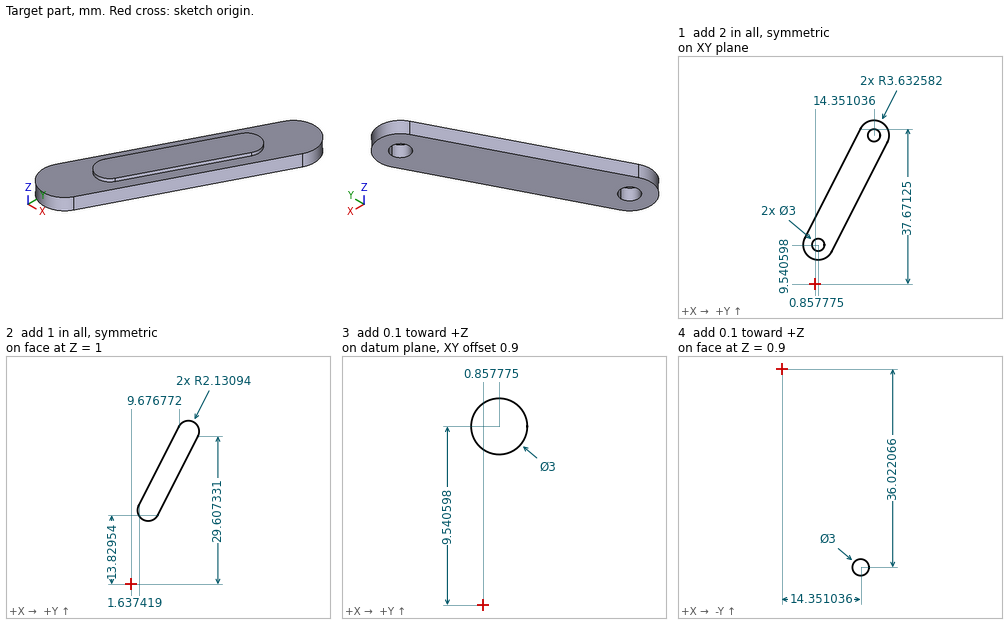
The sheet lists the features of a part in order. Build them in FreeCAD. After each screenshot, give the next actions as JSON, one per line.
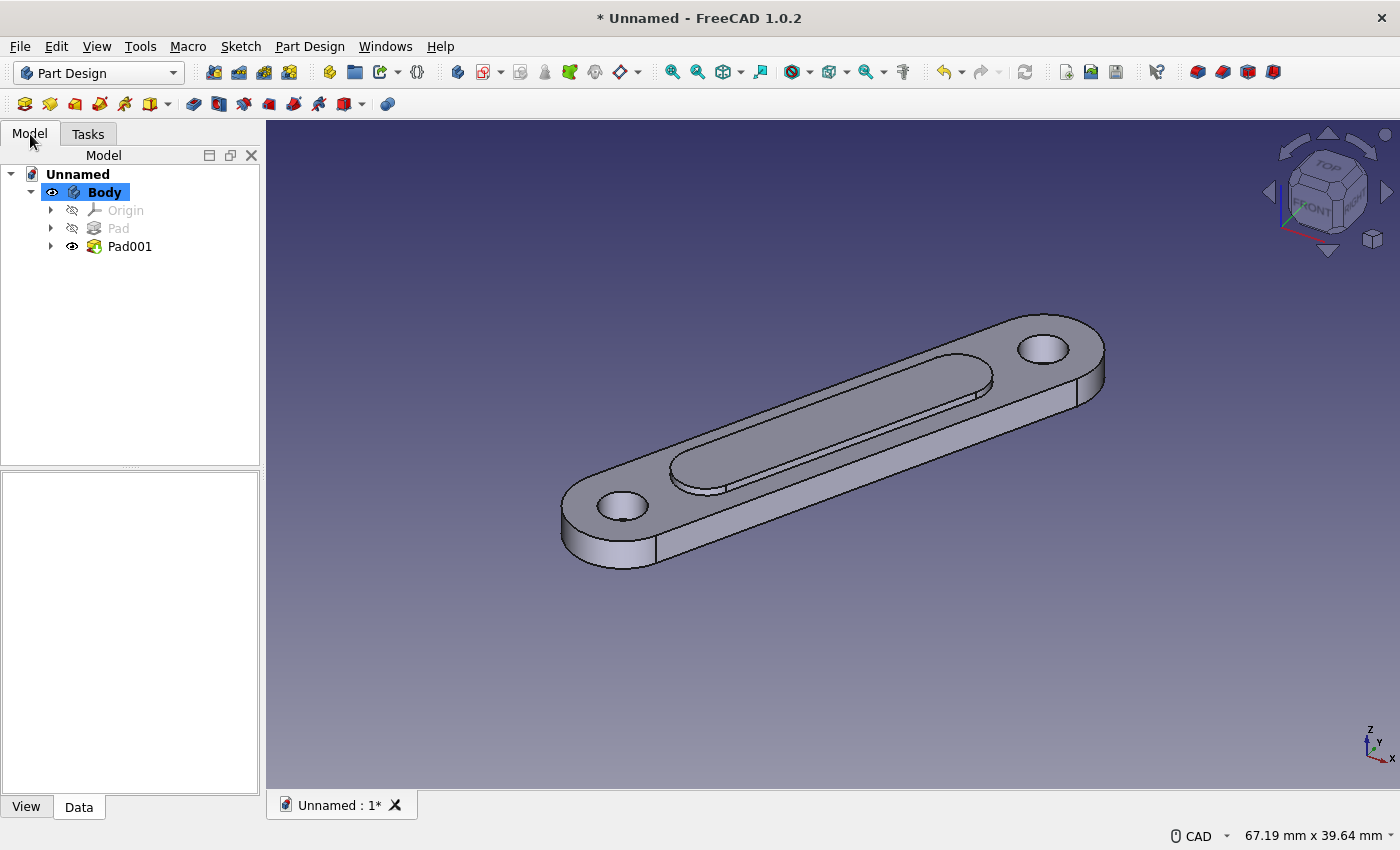
{"action": "left_click", "coordinate": [51, 210]}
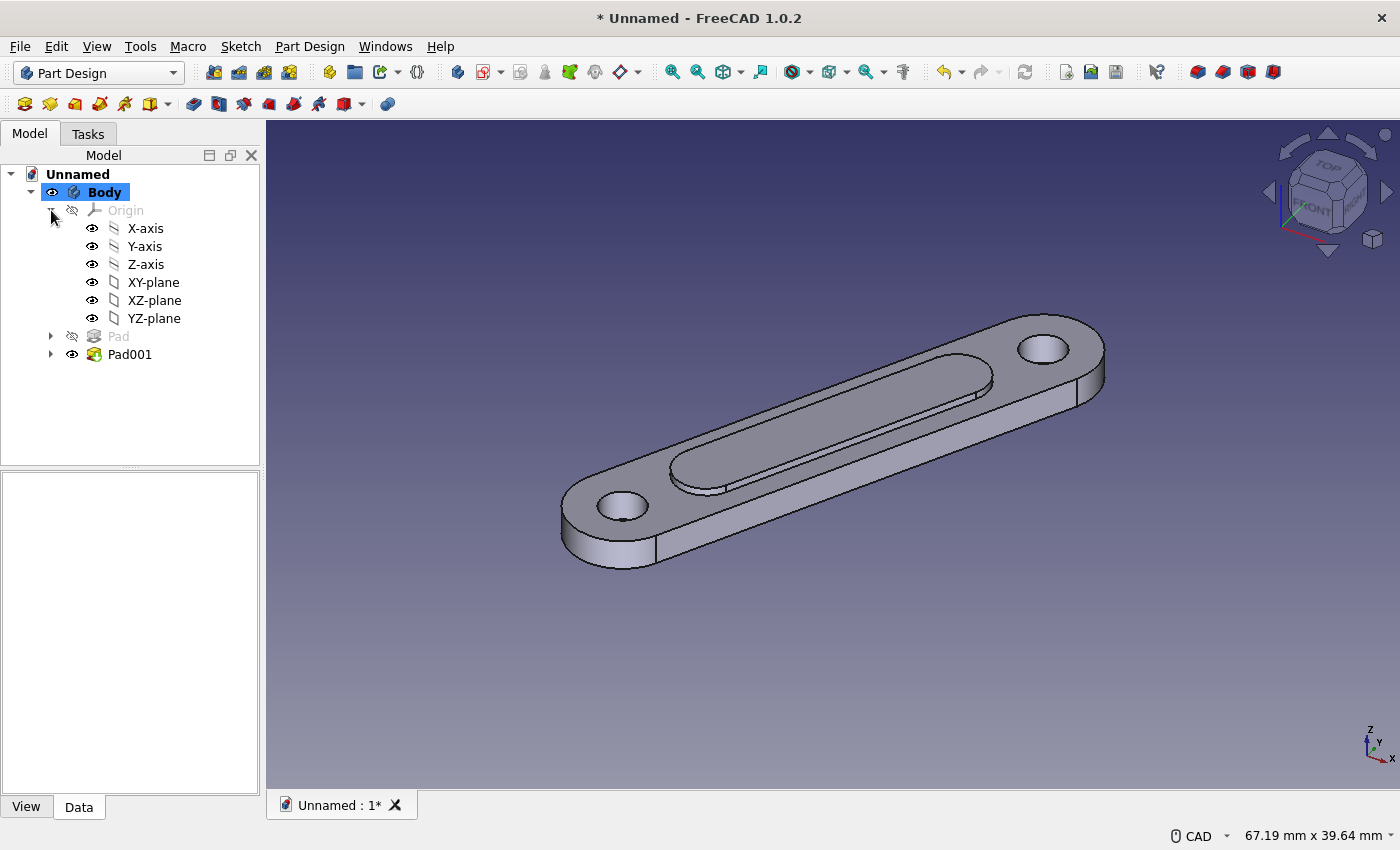
{"action": "left_click", "coordinate": [137, 282]}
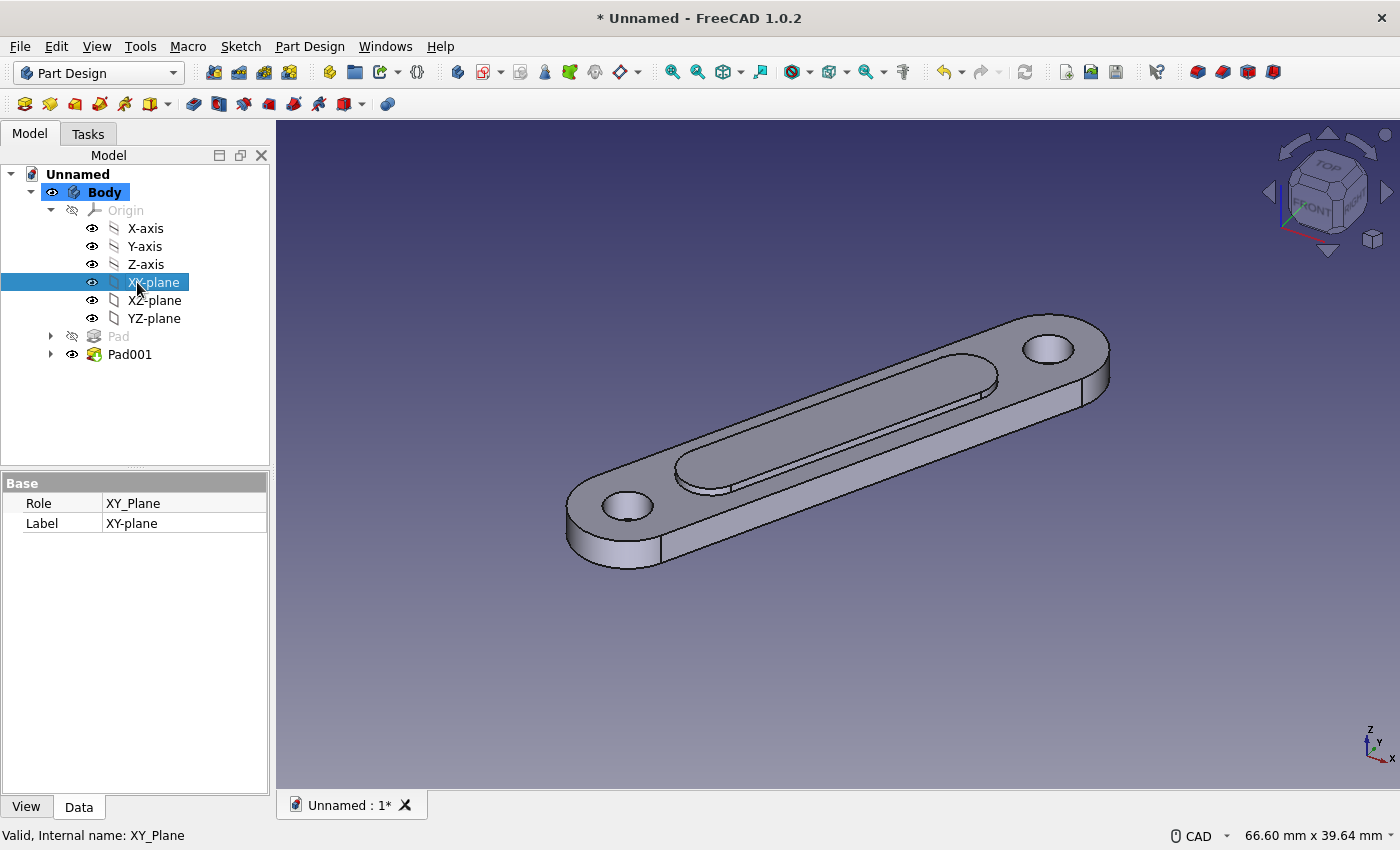
{"action": "left_click", "coordinate": [620, 72]}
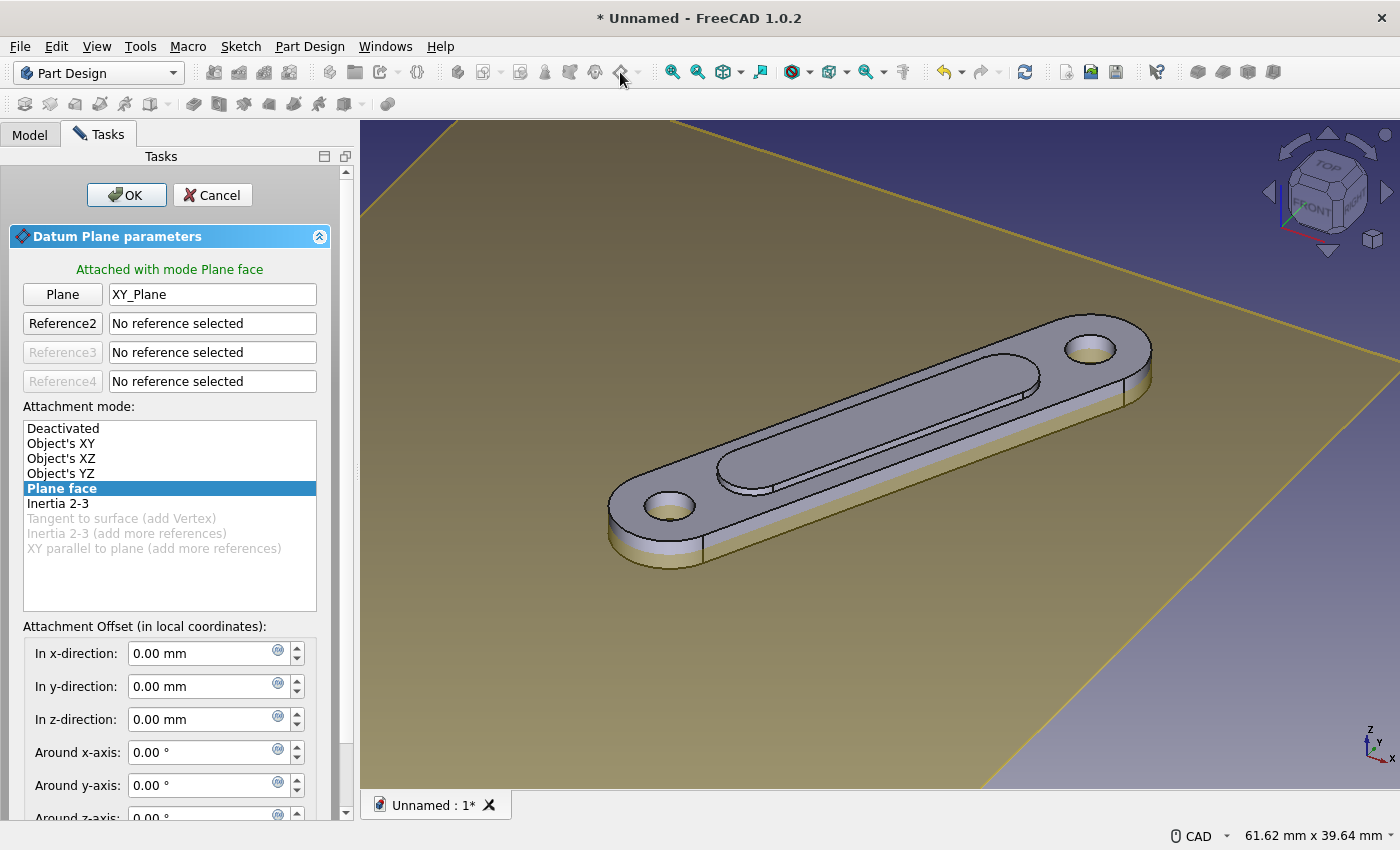
{"action": "triple_click", "coordinate": [210, 720]}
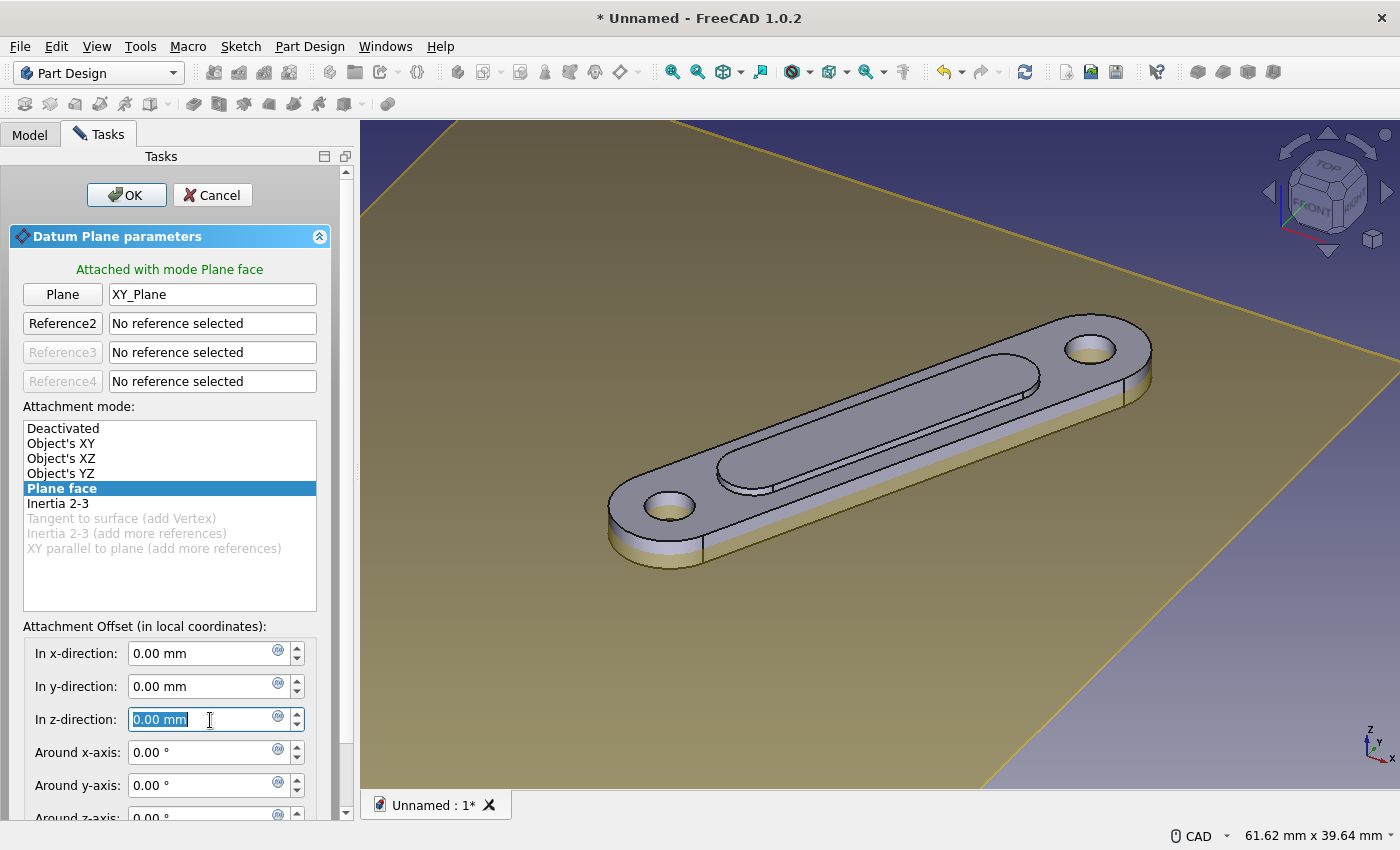
{"action": "type", "text": "0.9"}
{"action": "key", "text": "Tab"}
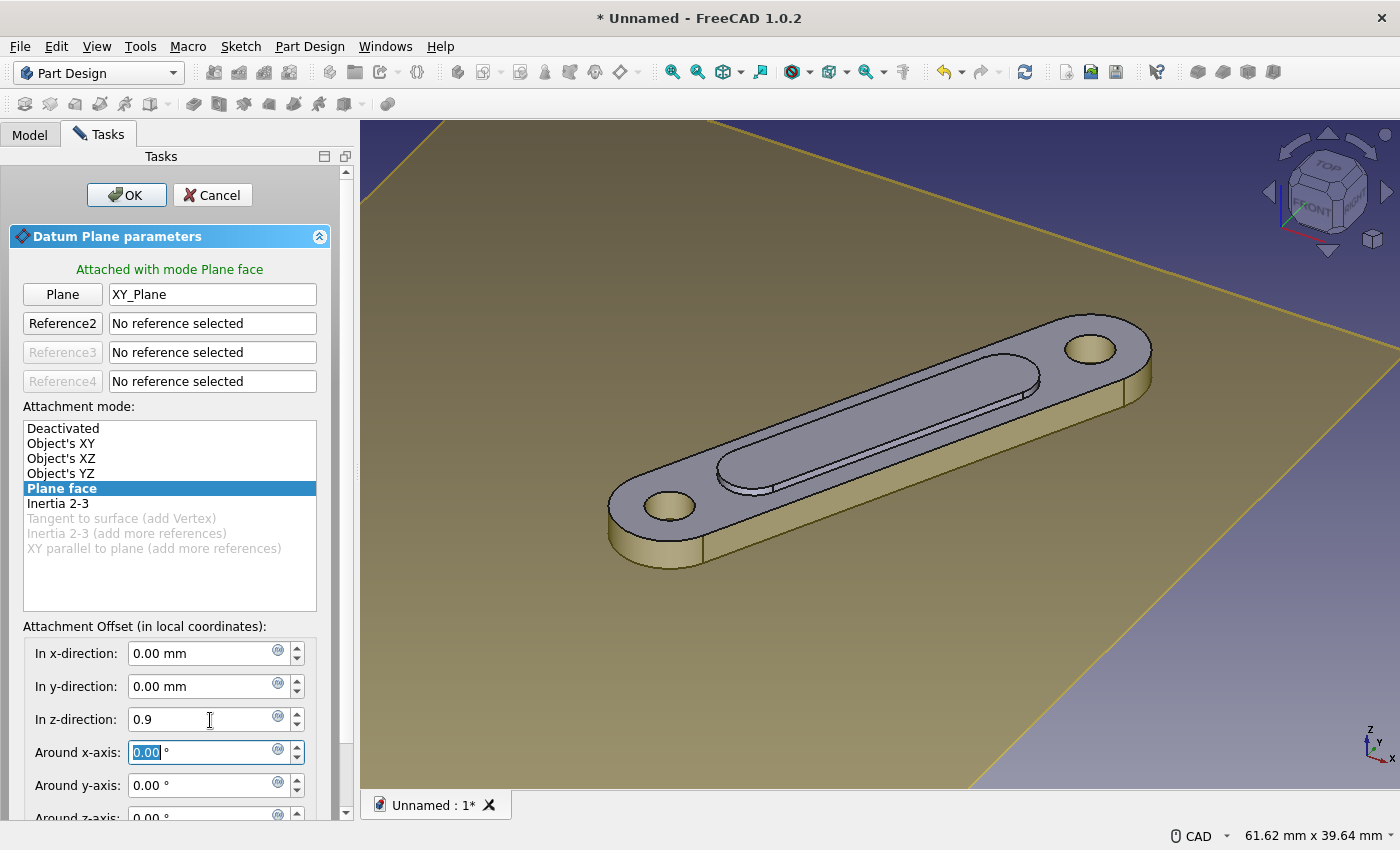
{"action": "left_click", "coordinate": [127, 195]}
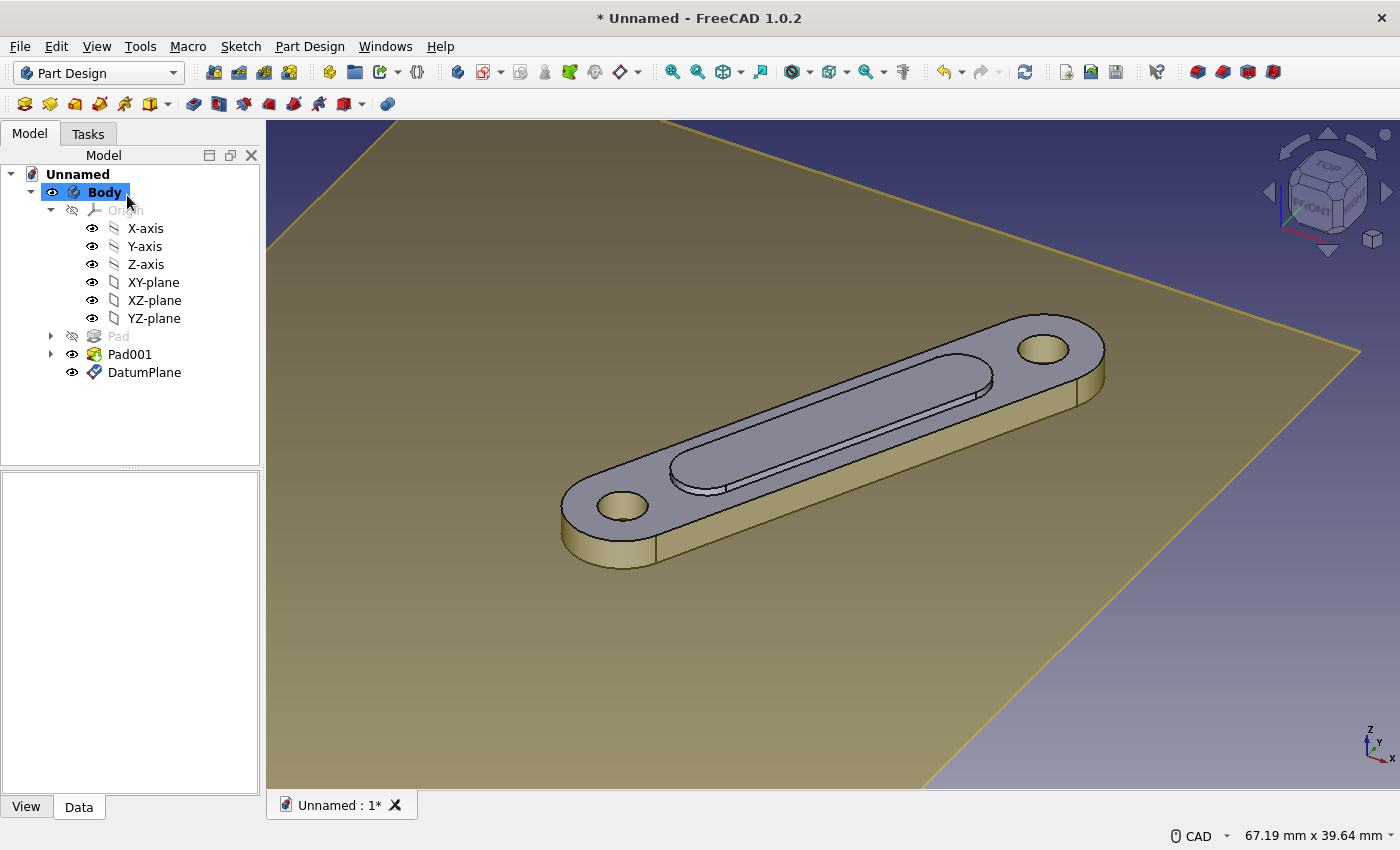
{"action": "left_click", "coordinate": [117, 372]}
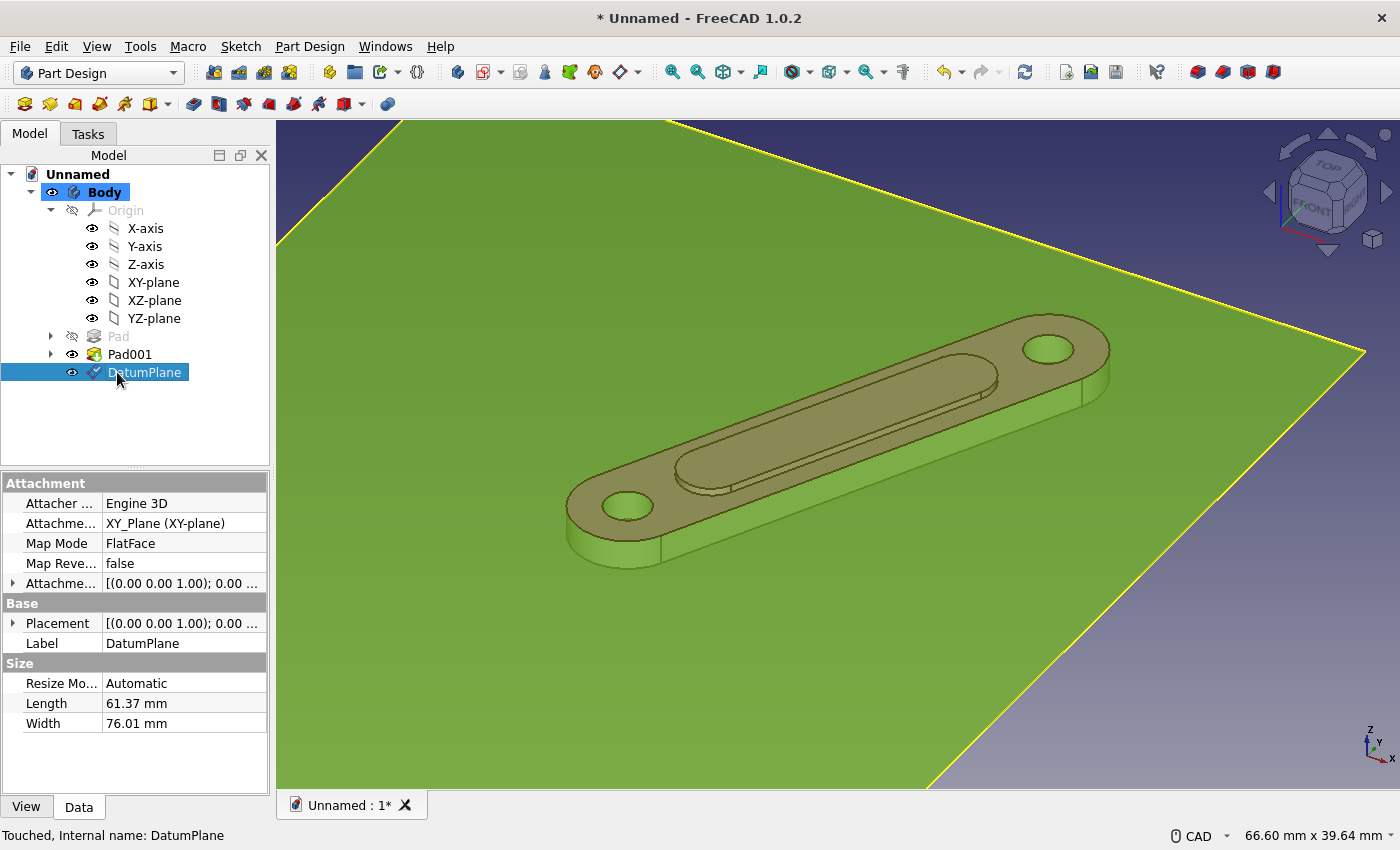
{"action": "left_click", "coordinate": [482, 72]}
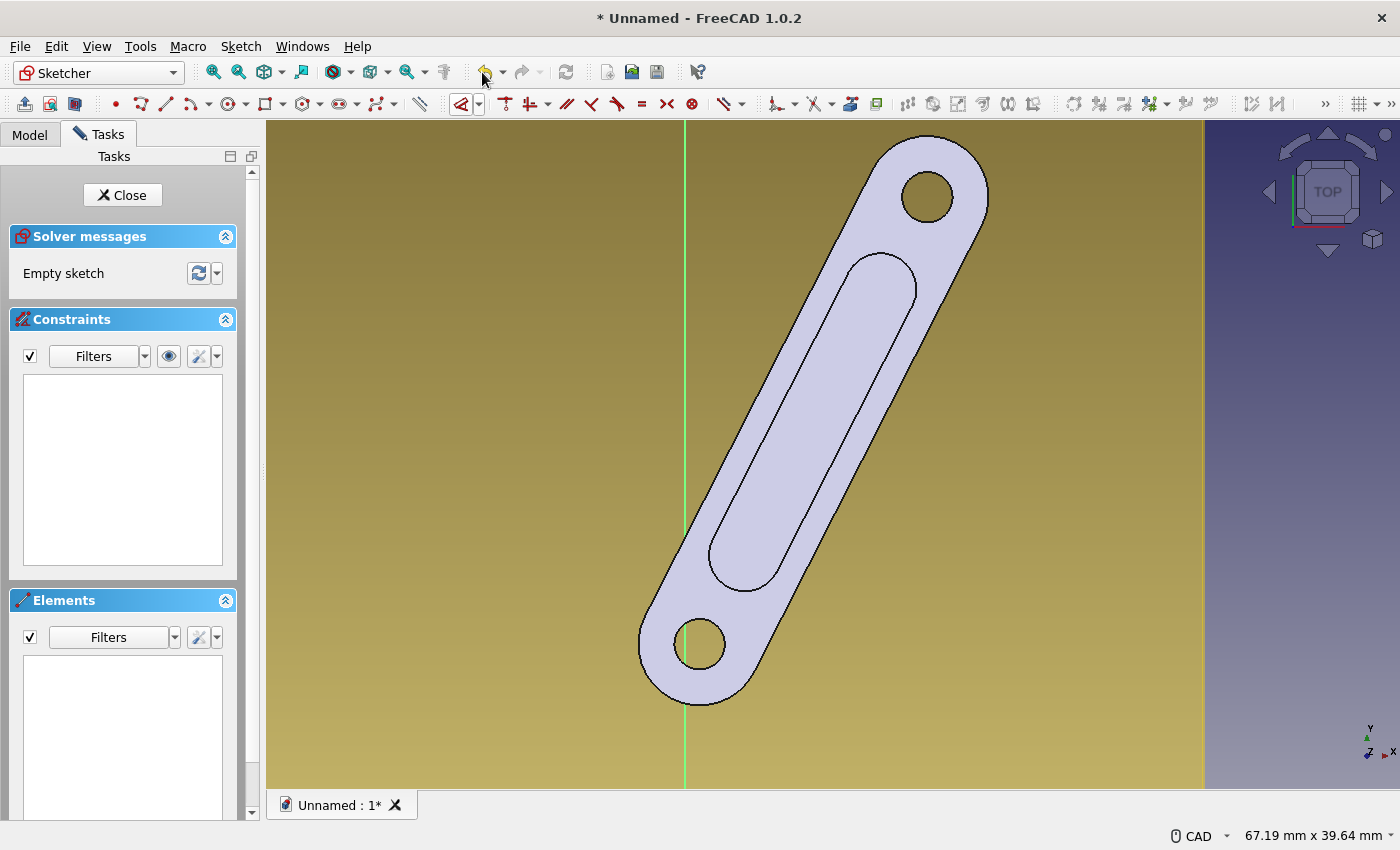
{"action": "left_click", "coordinate": [75, 104]}